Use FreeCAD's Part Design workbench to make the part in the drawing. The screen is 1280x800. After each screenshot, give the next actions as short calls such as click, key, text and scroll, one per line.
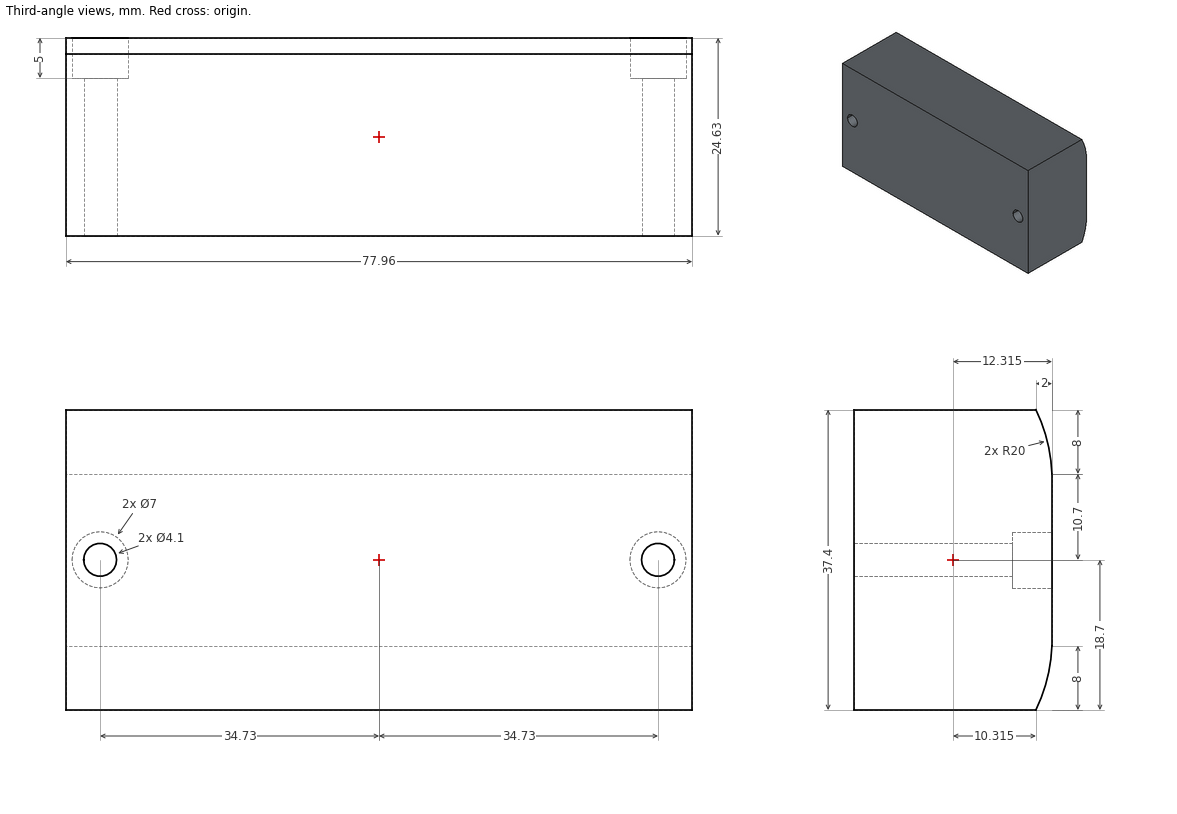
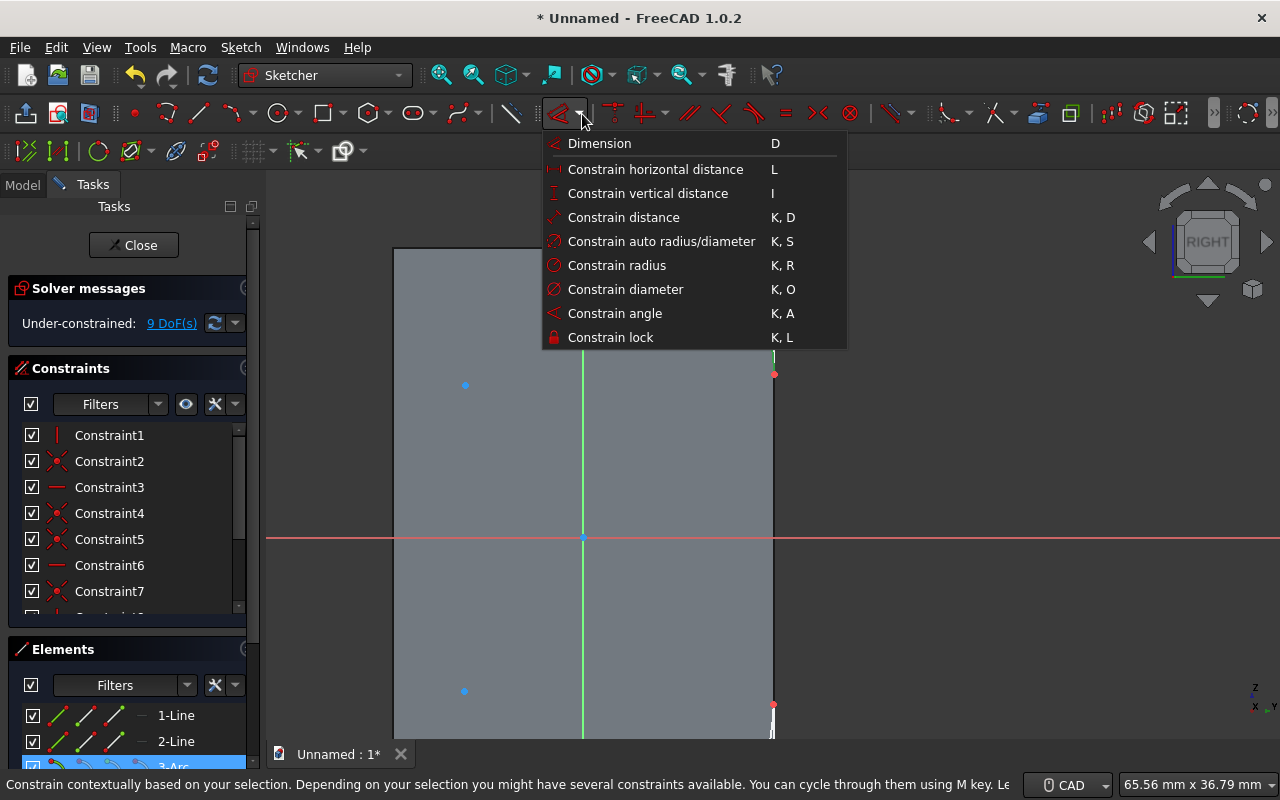
click(695, 265)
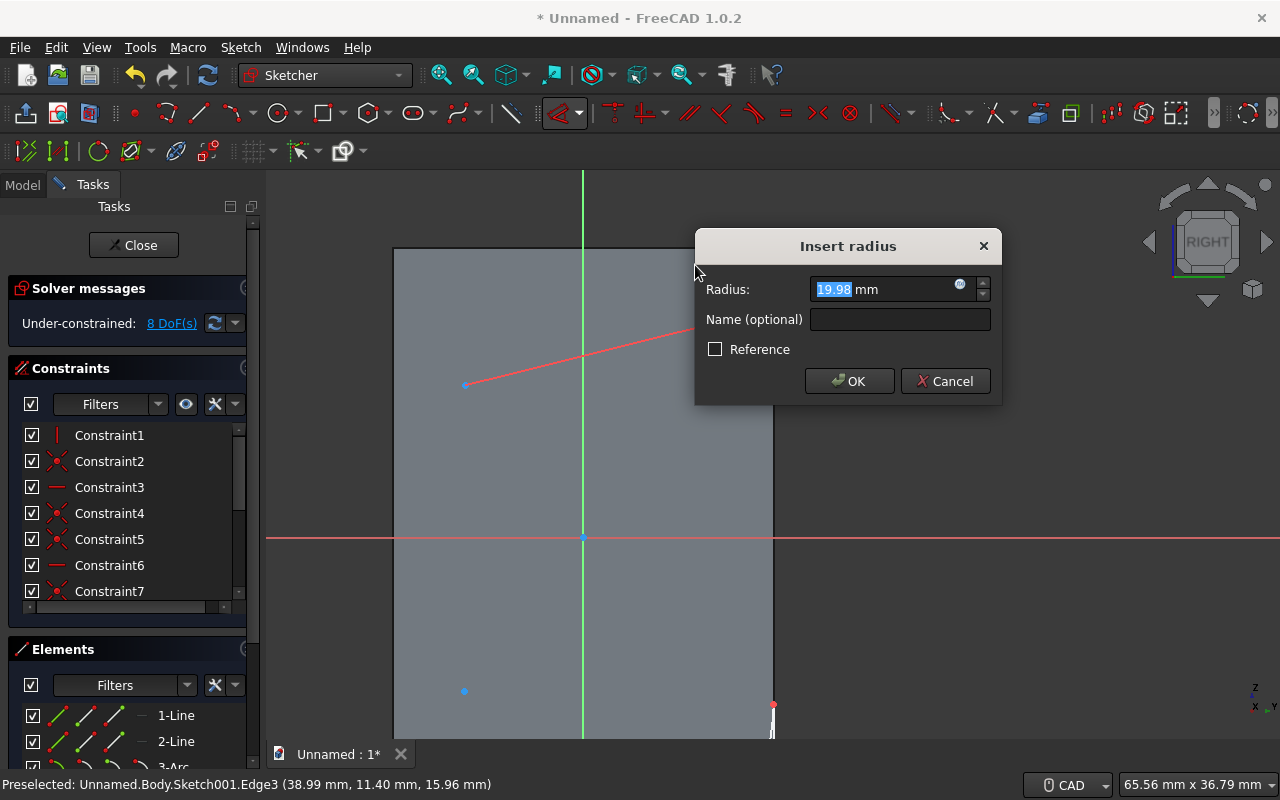
text(20)
key(Return)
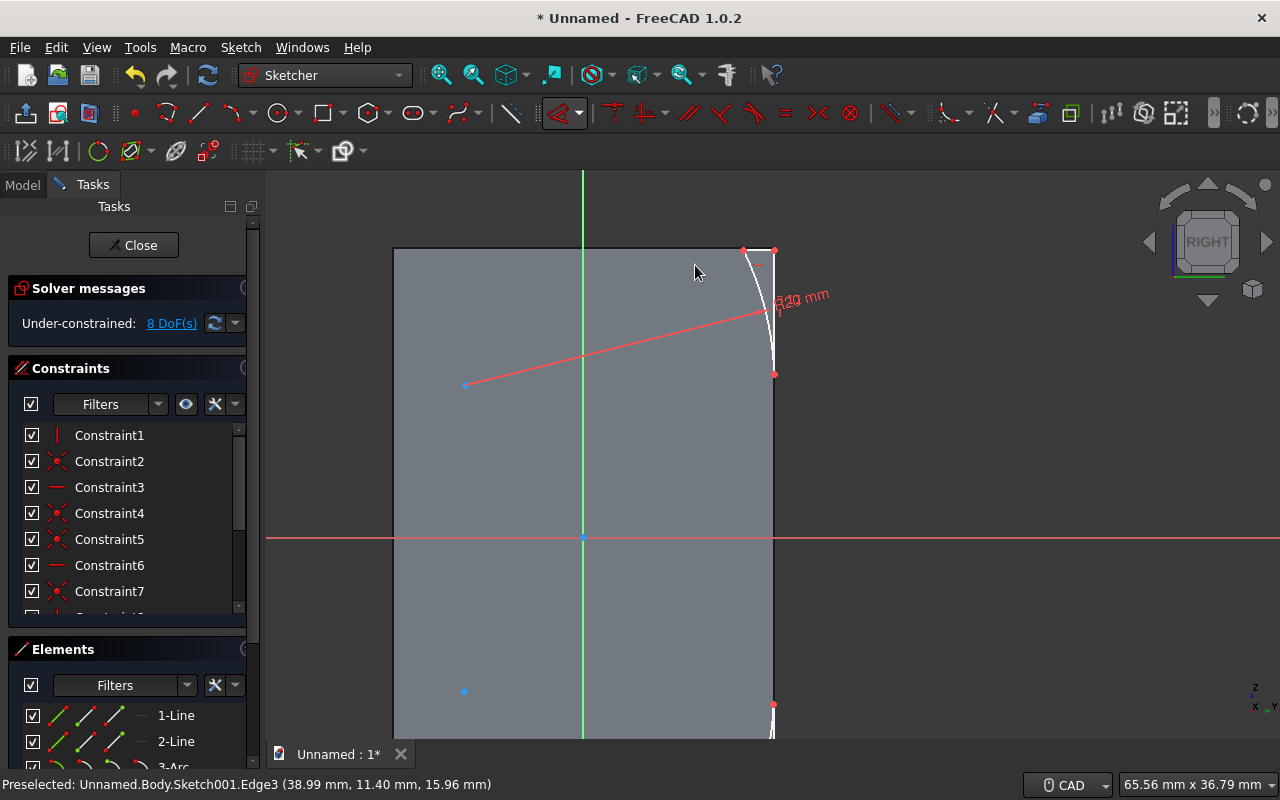
click(774, 287)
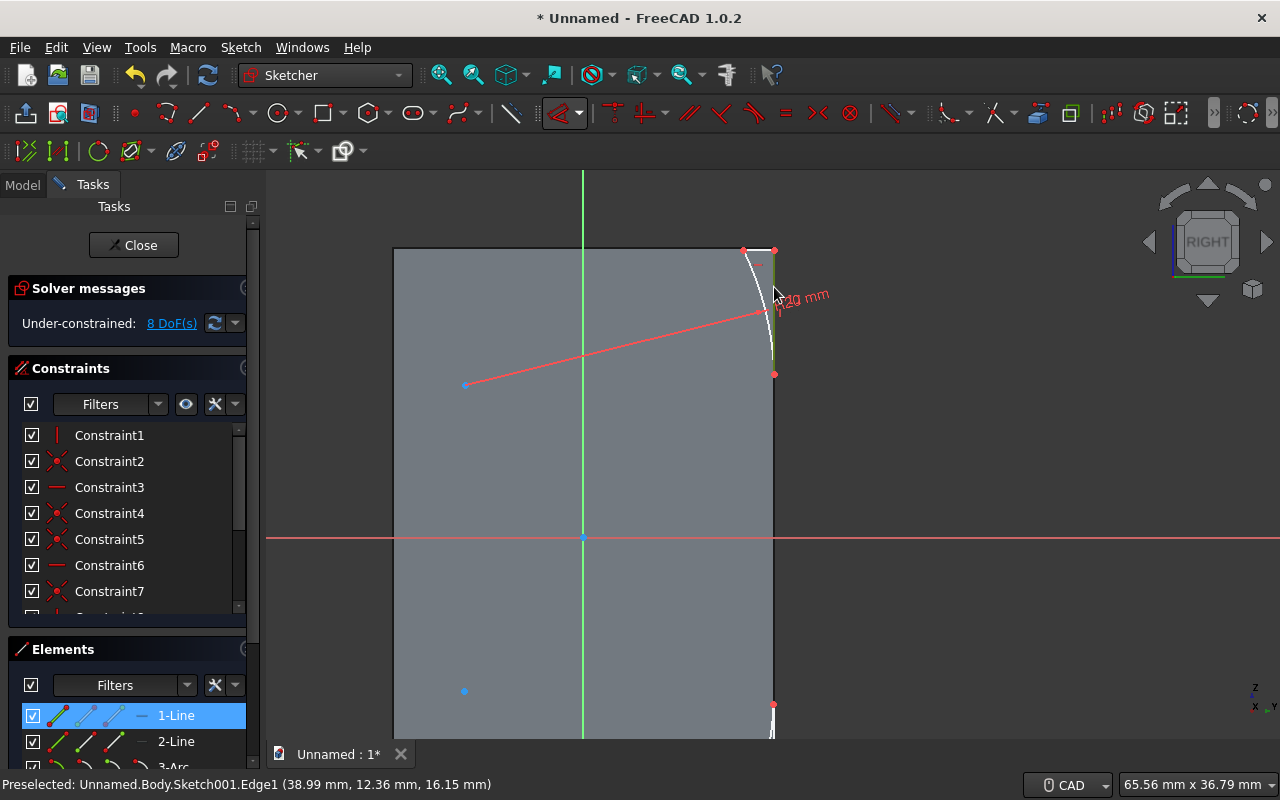
click(582, 114)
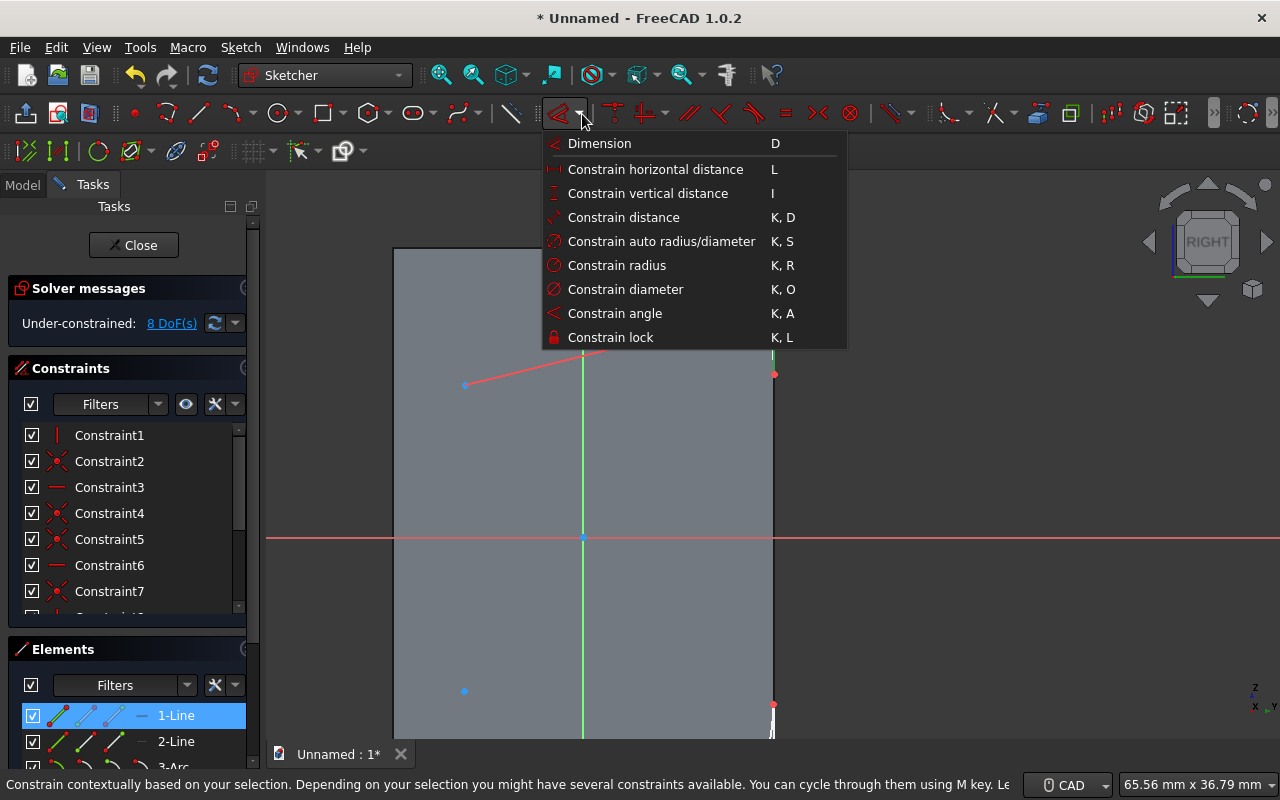
click(695, 193)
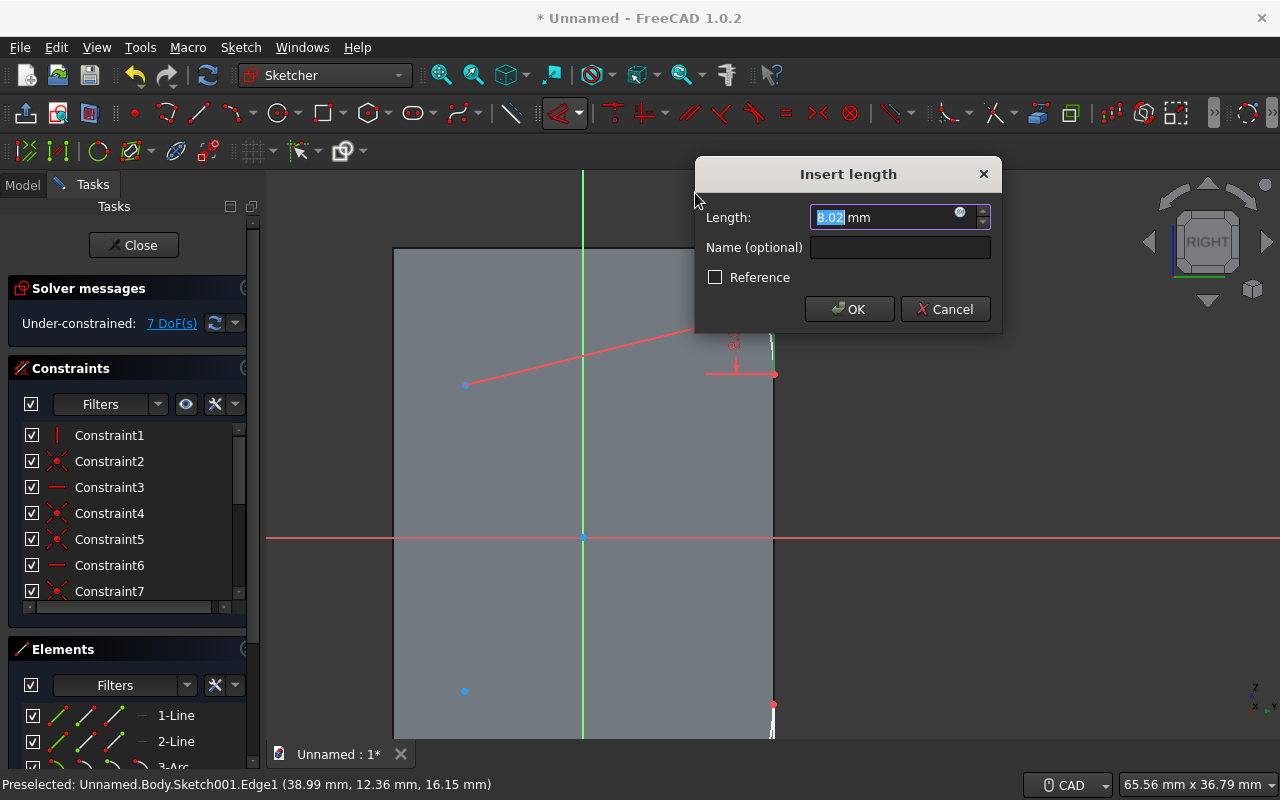
text(8)
key(Return)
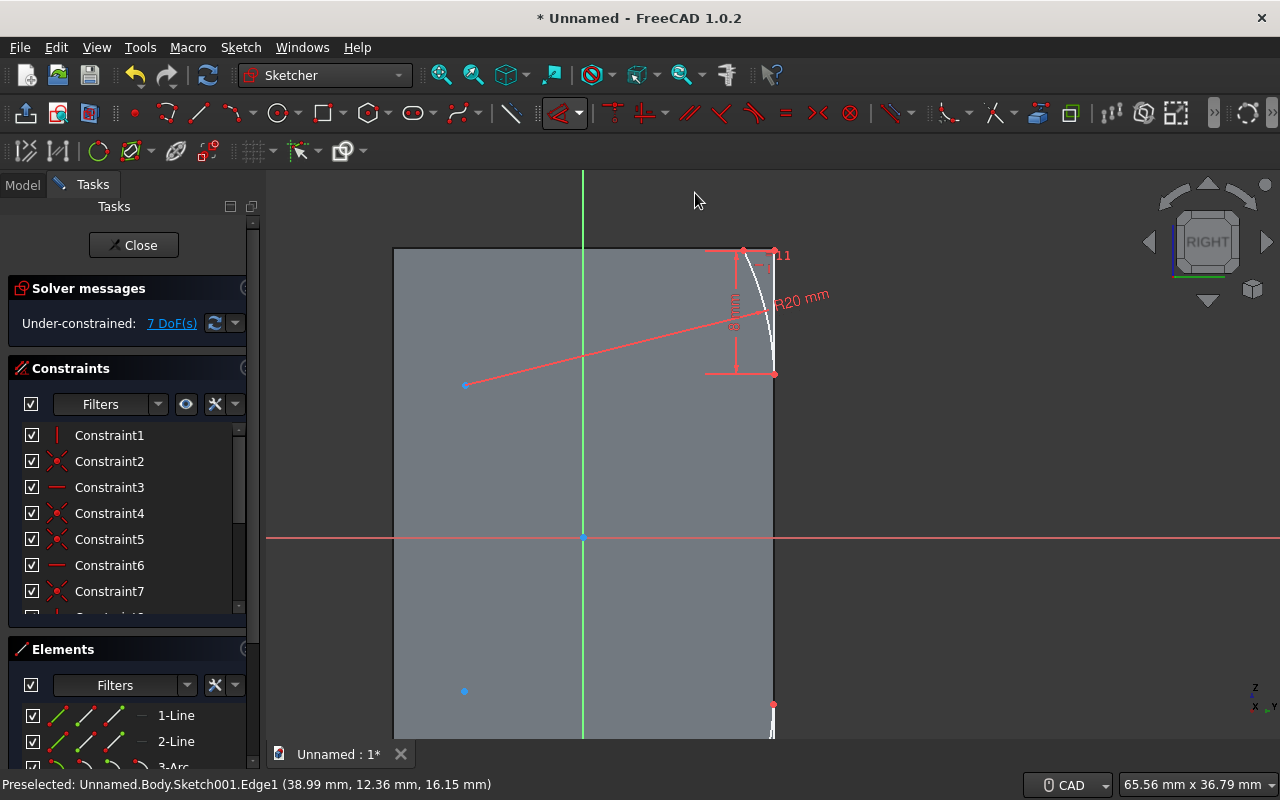
scroll(765, 251, up, 3)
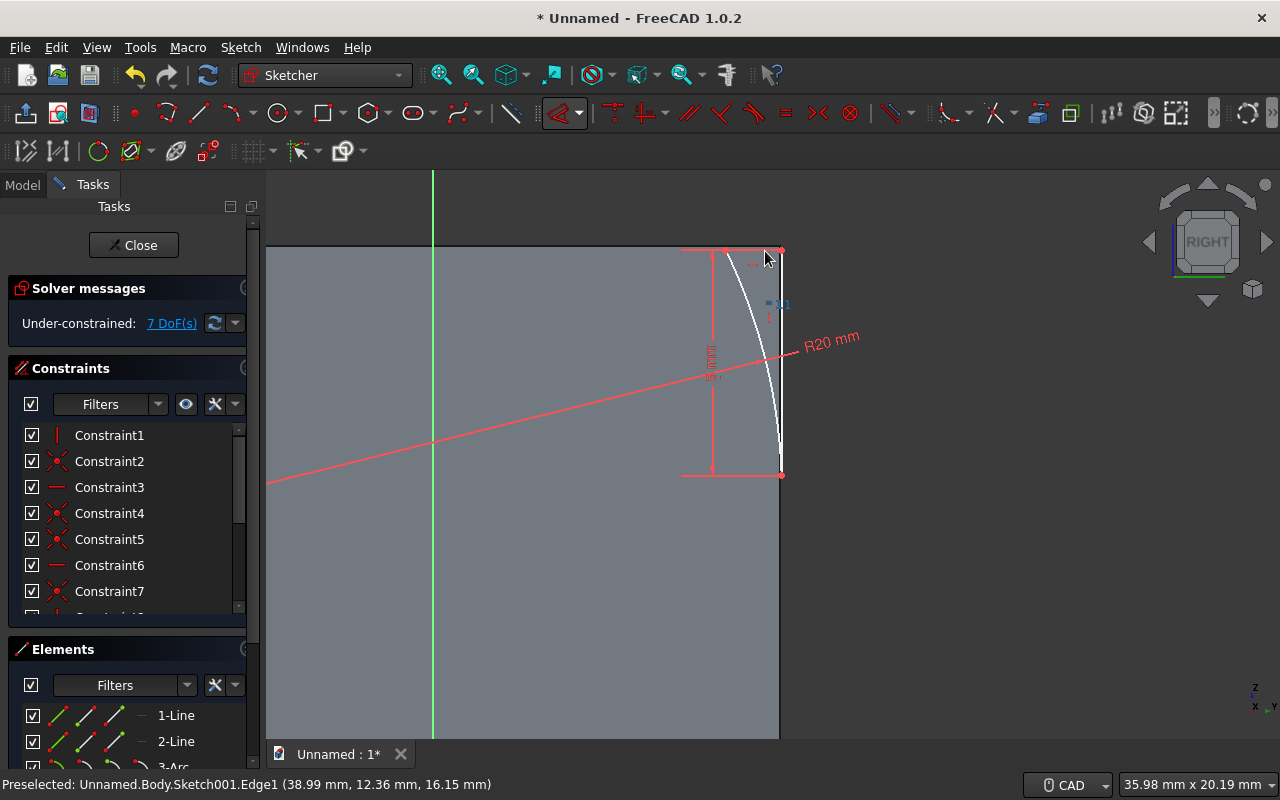
click(765, 250)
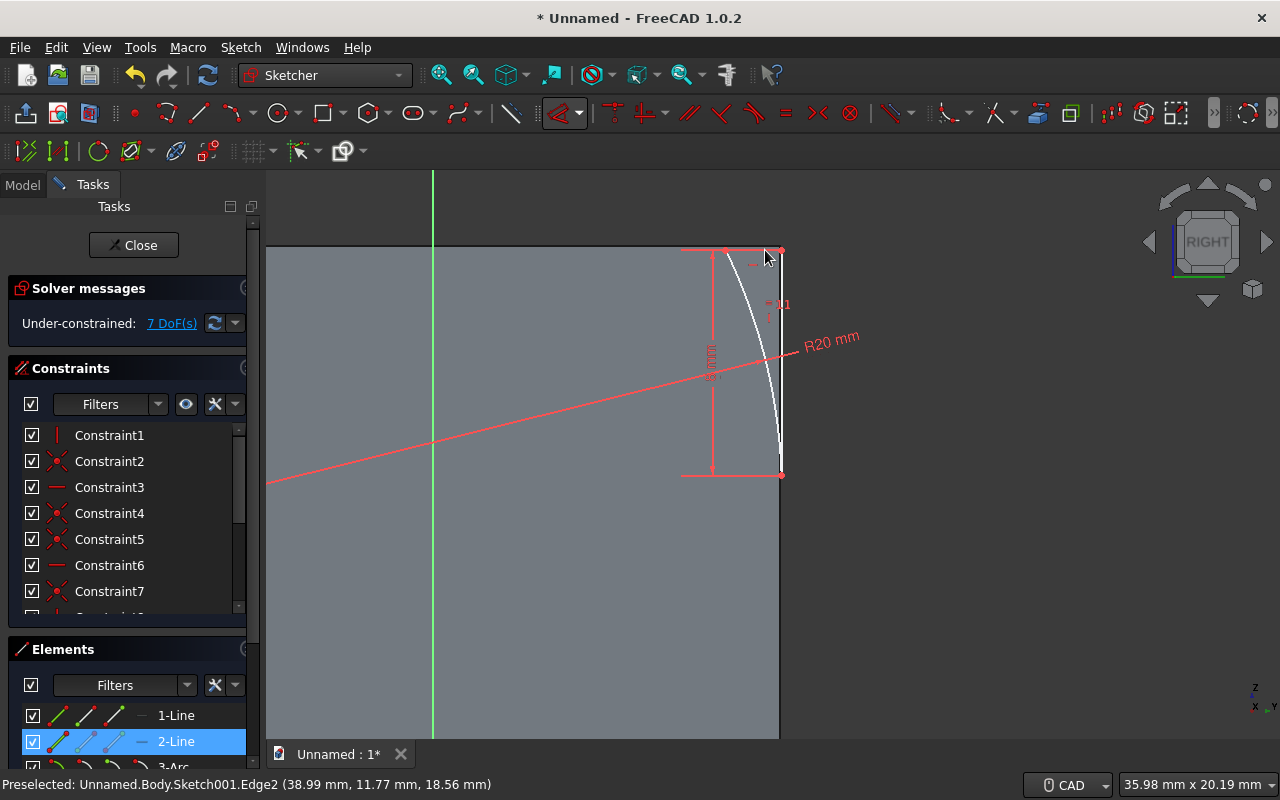
key(l)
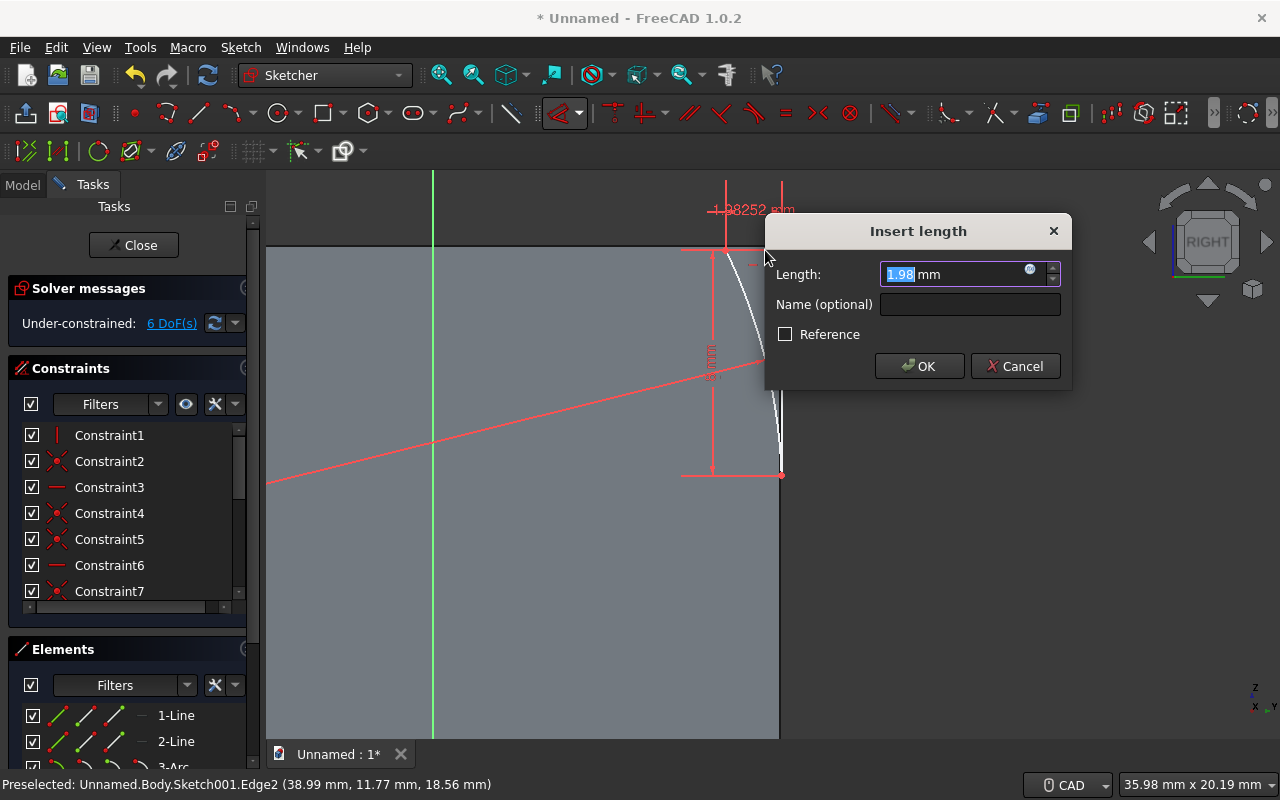
text(2)
key(Return)